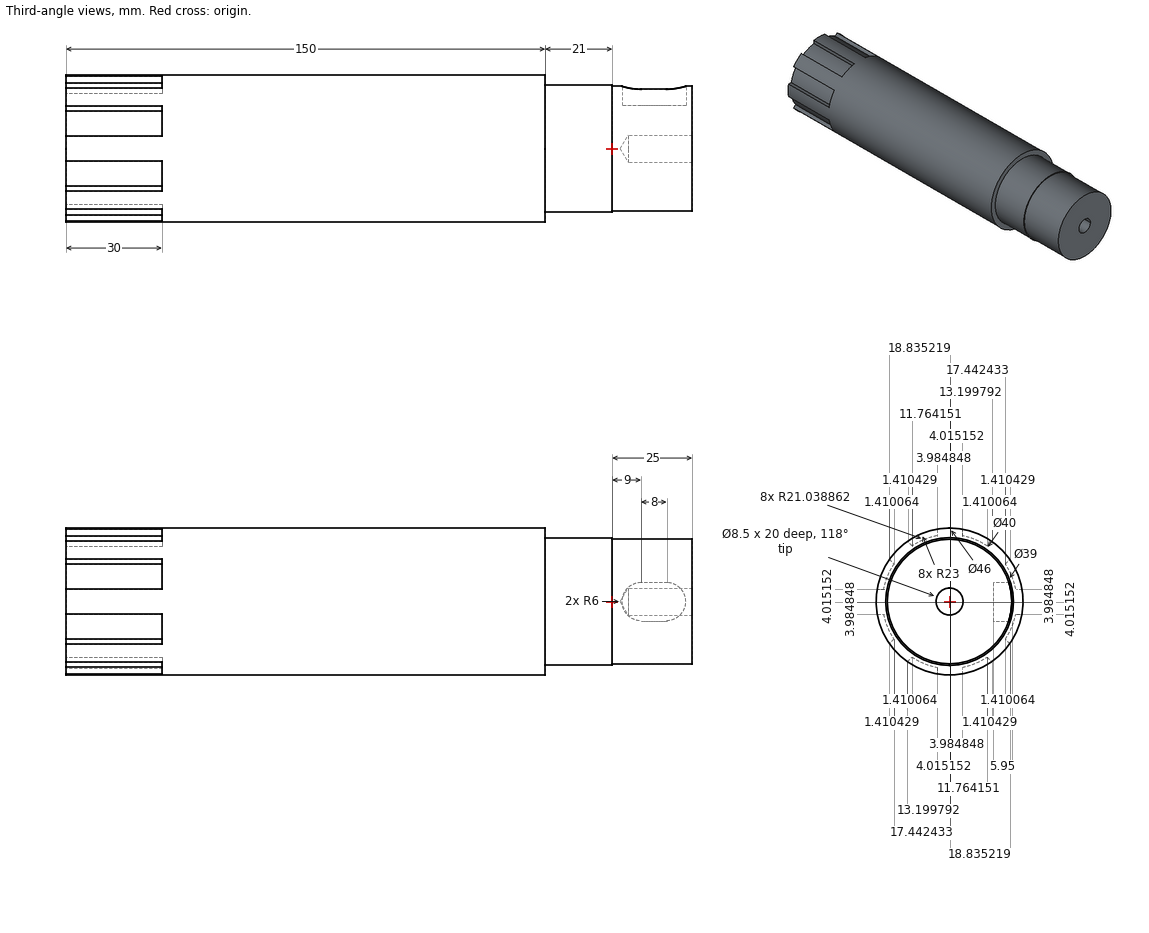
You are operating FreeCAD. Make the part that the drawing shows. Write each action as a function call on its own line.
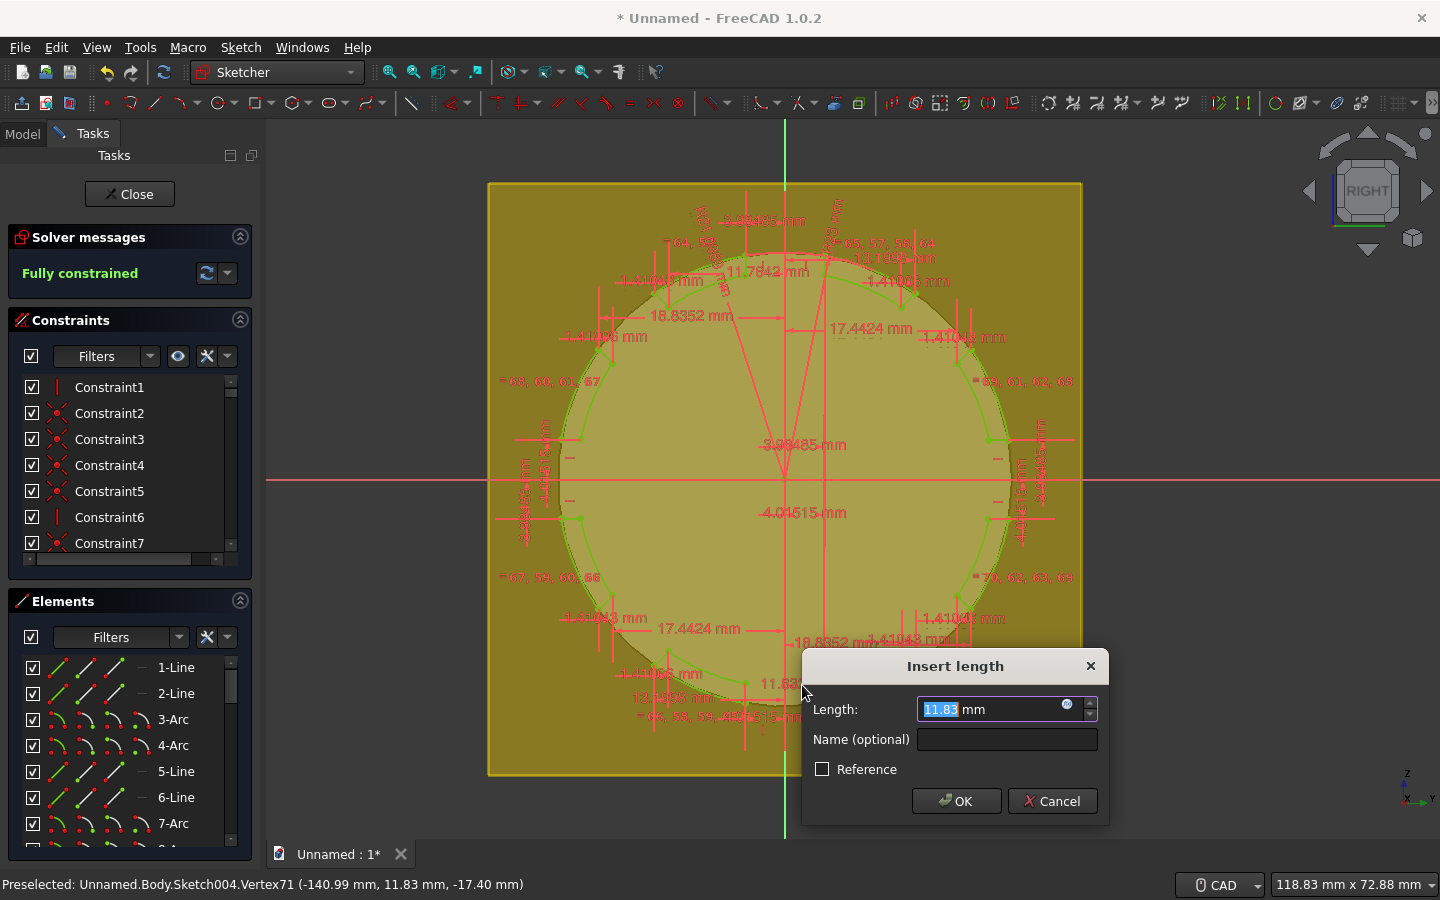
text(11.764151)
key(Return)
key(Escape)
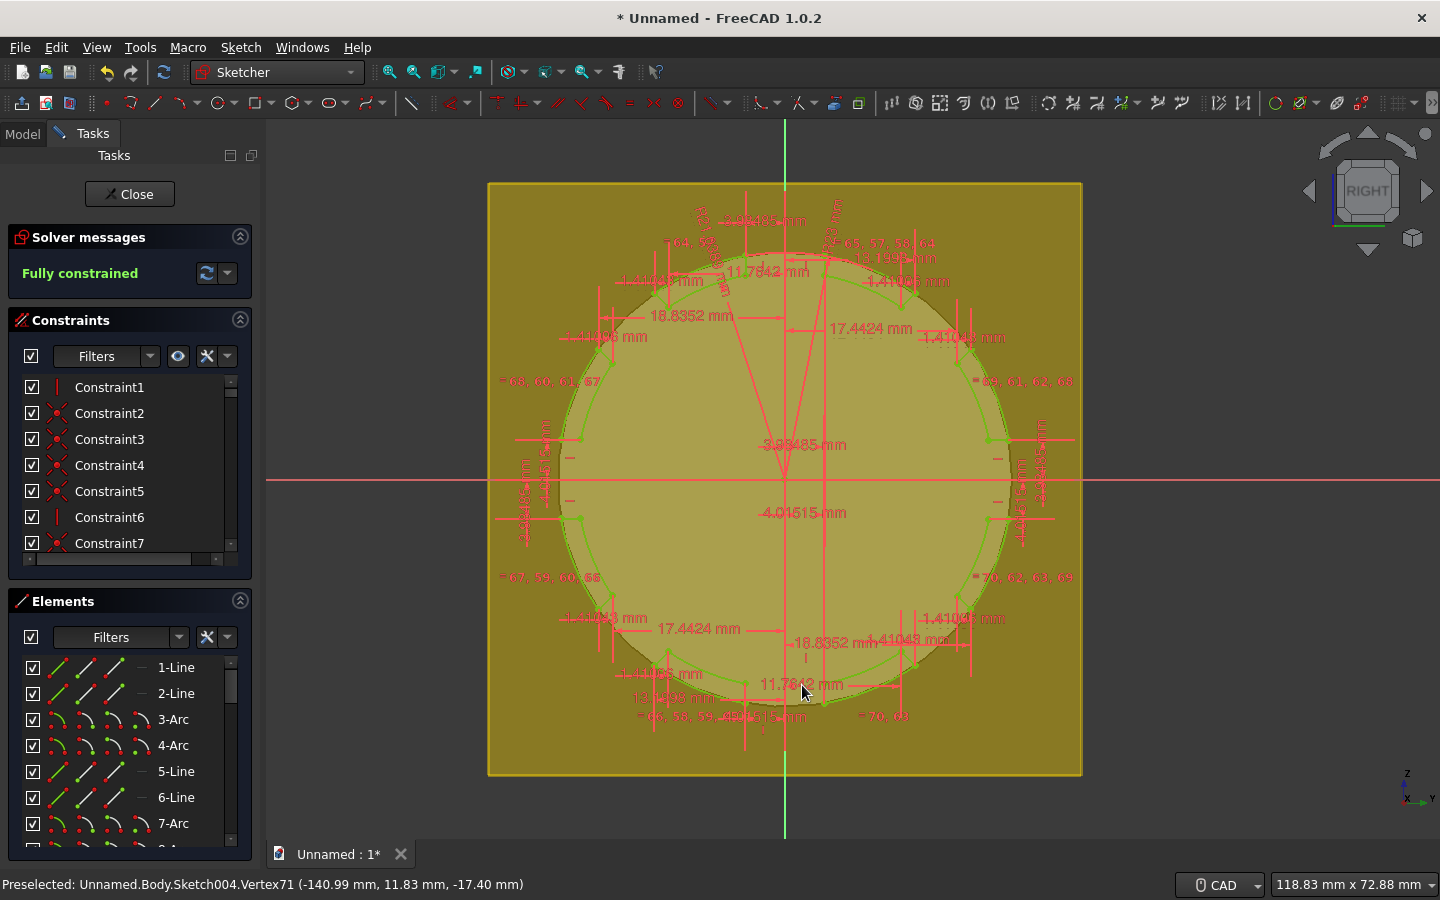
click(130, 194)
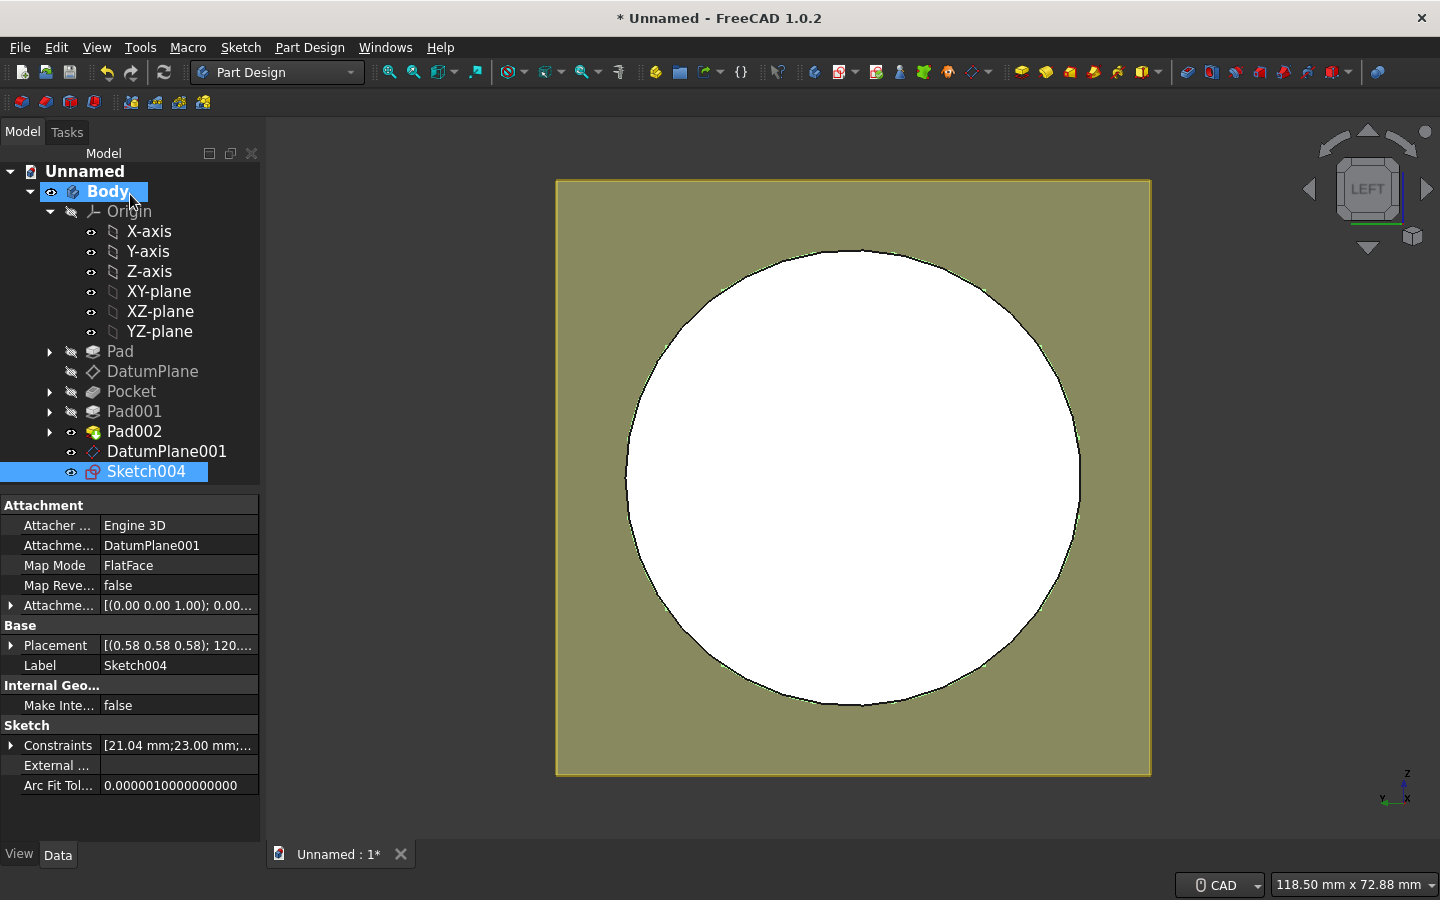
click(1188, 72)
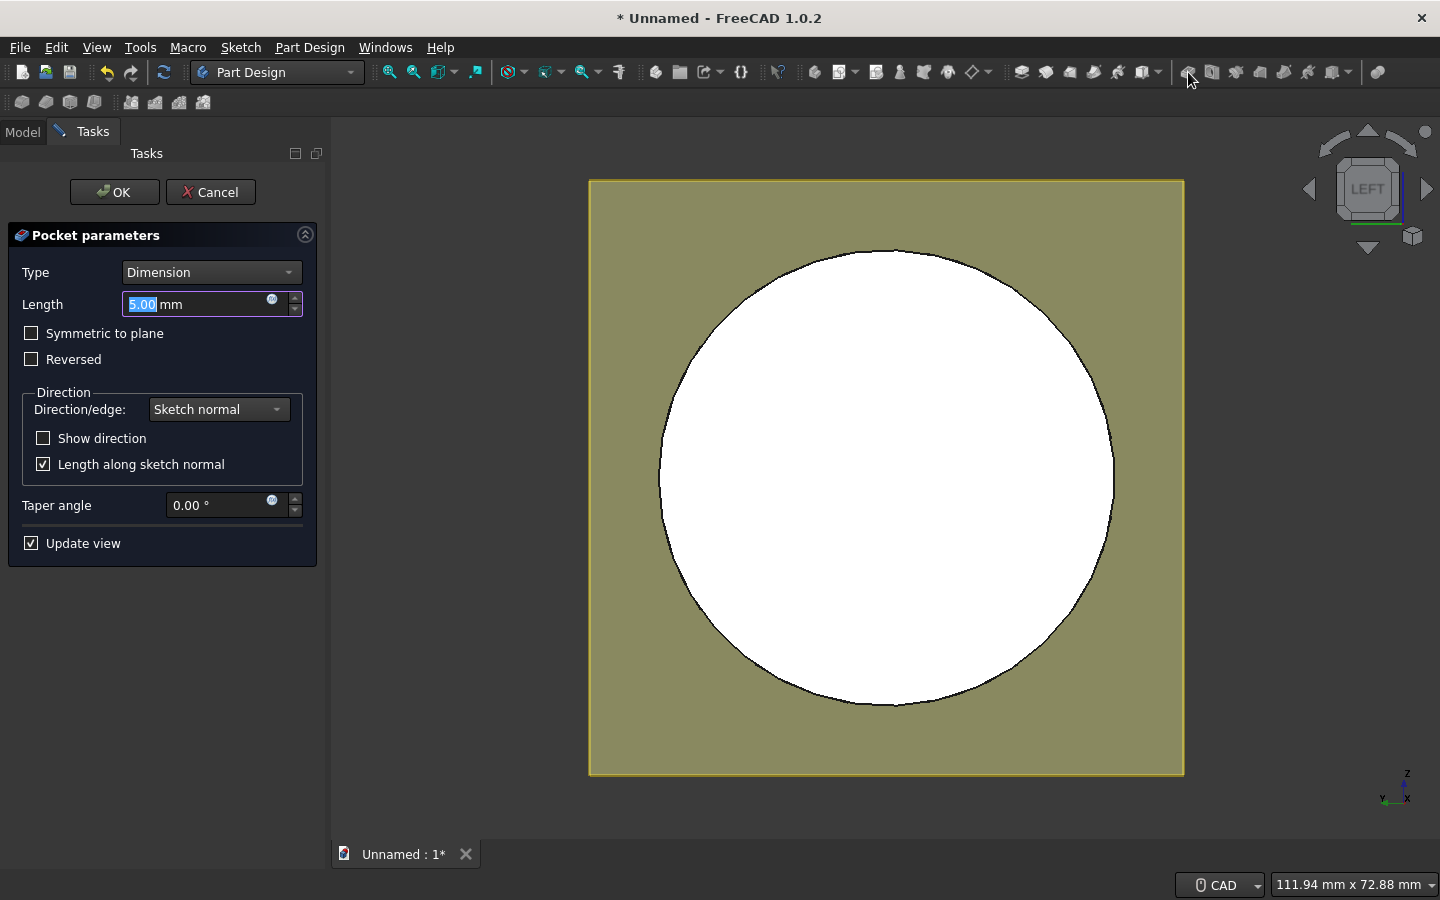
text(30)
key(Tab)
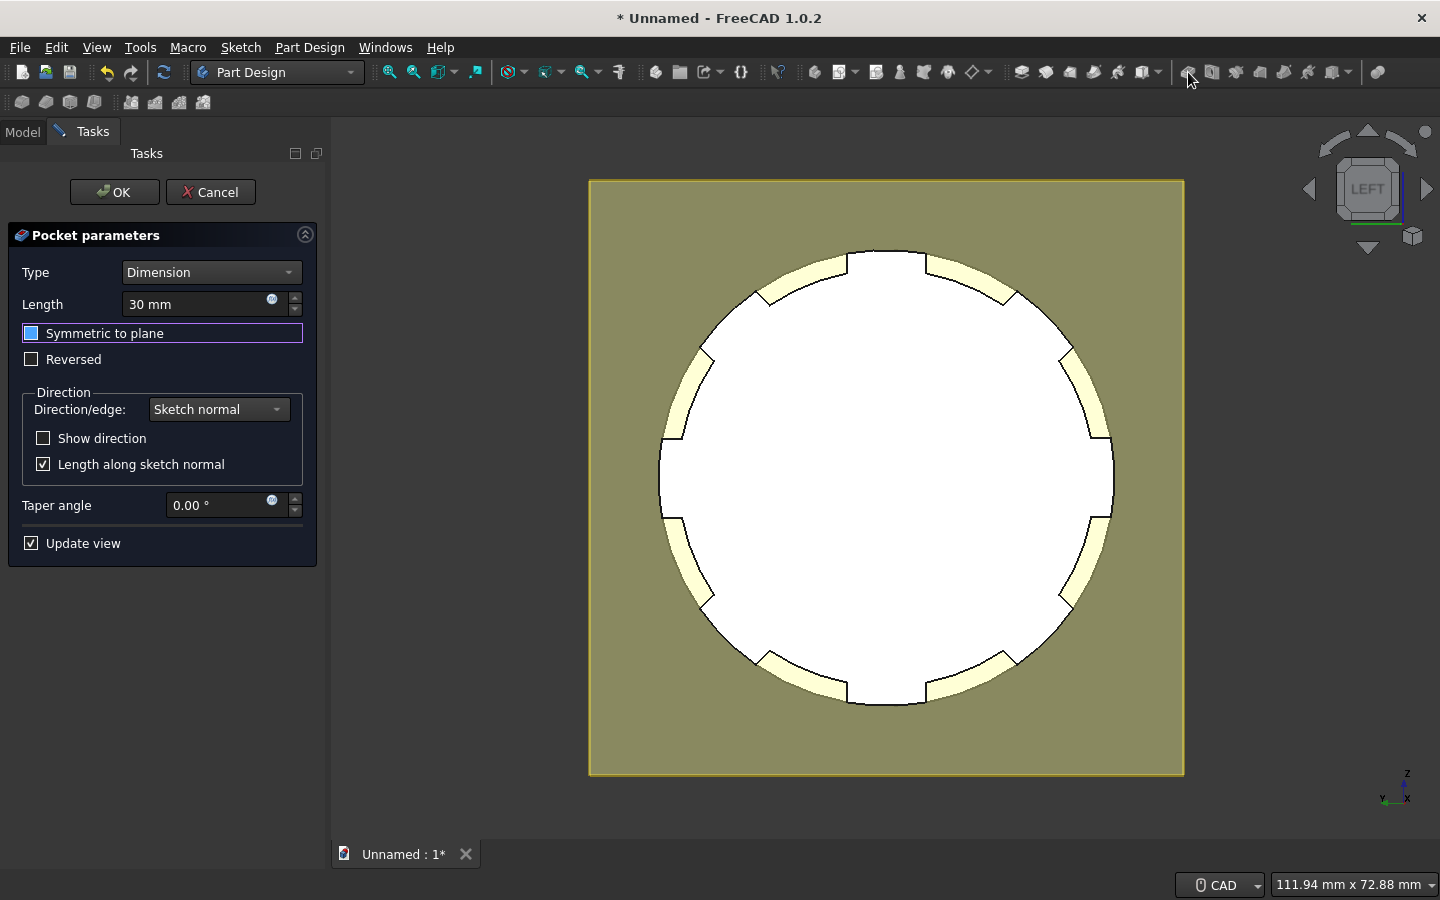
click(115, 192)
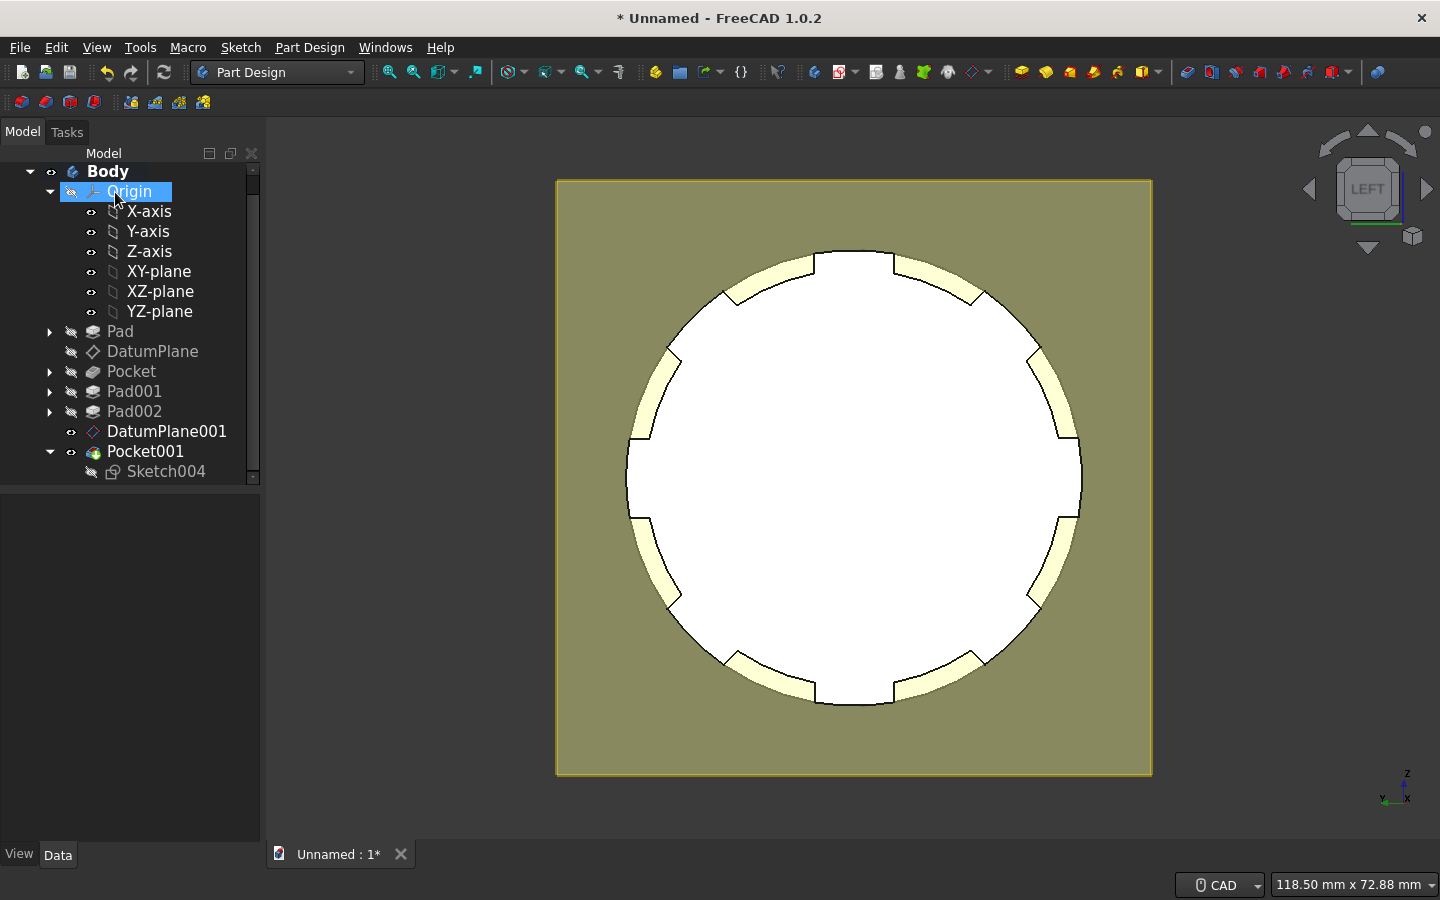
click(116, 432)
key(space)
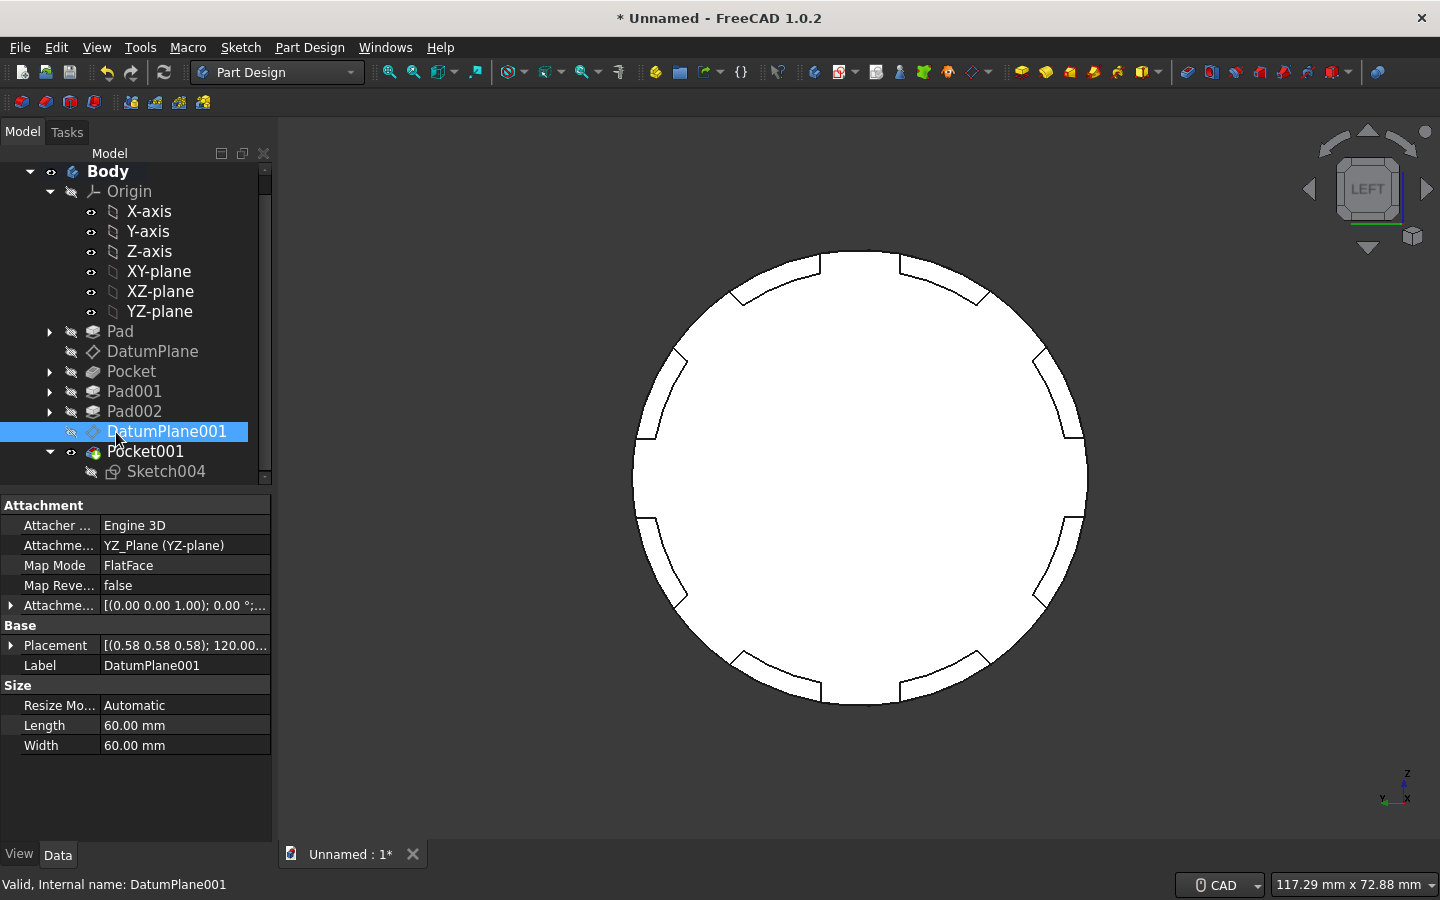
key(0)